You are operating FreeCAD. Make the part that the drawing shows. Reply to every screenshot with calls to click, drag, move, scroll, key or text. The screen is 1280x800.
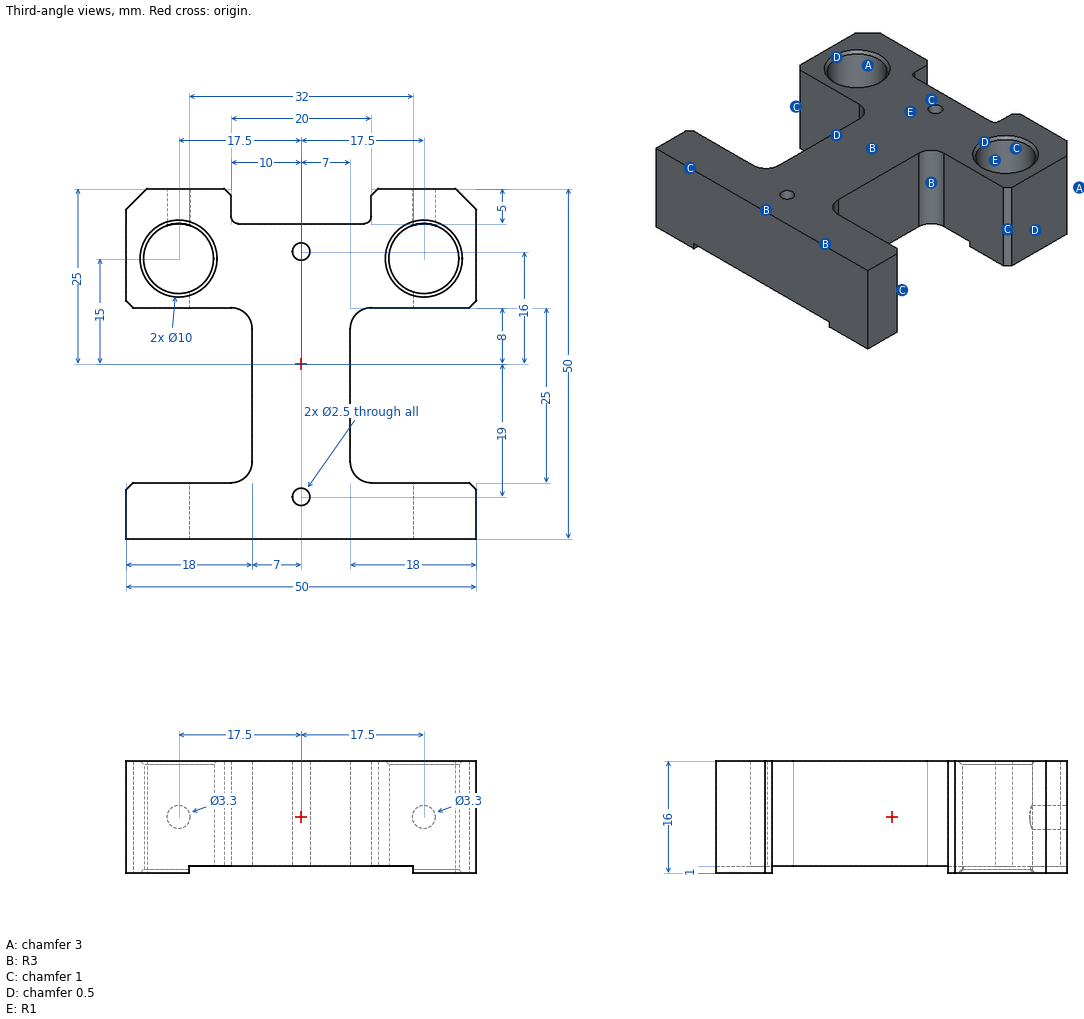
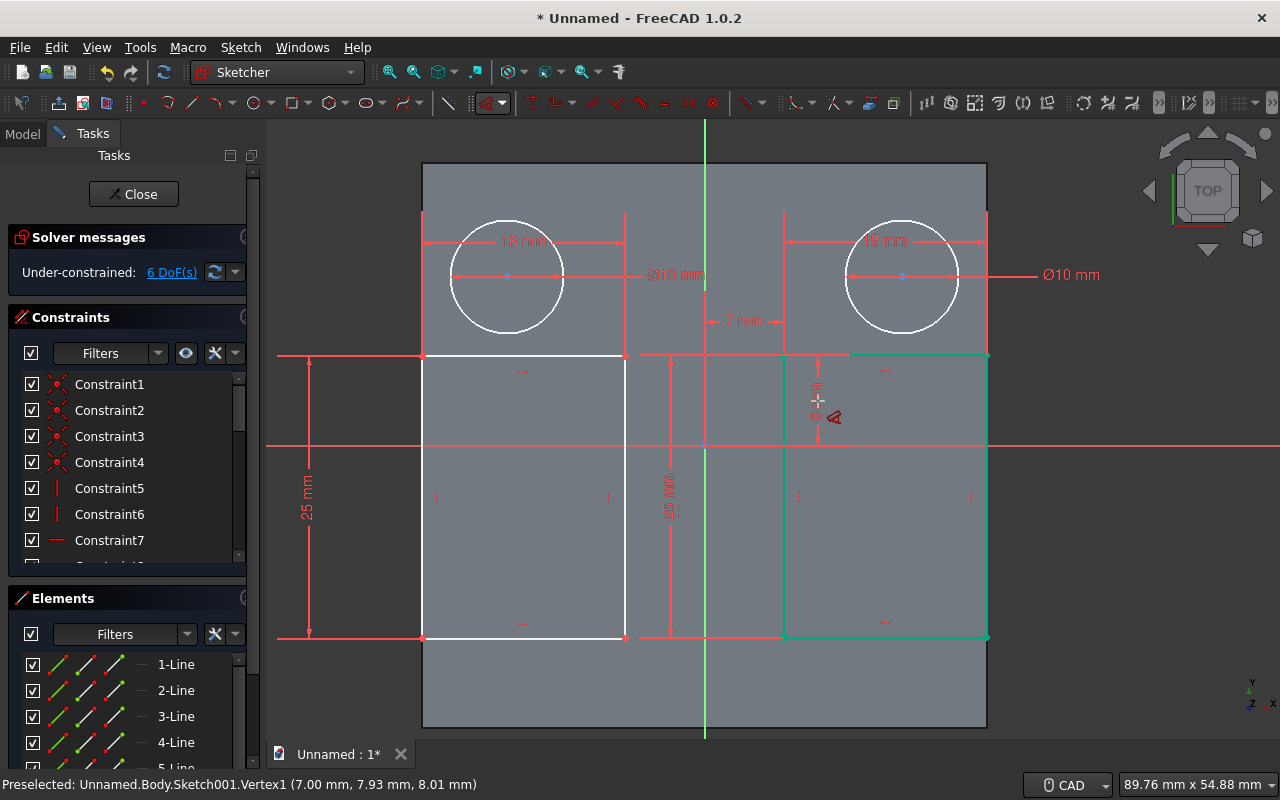
click(422, 356)
click(388, 401)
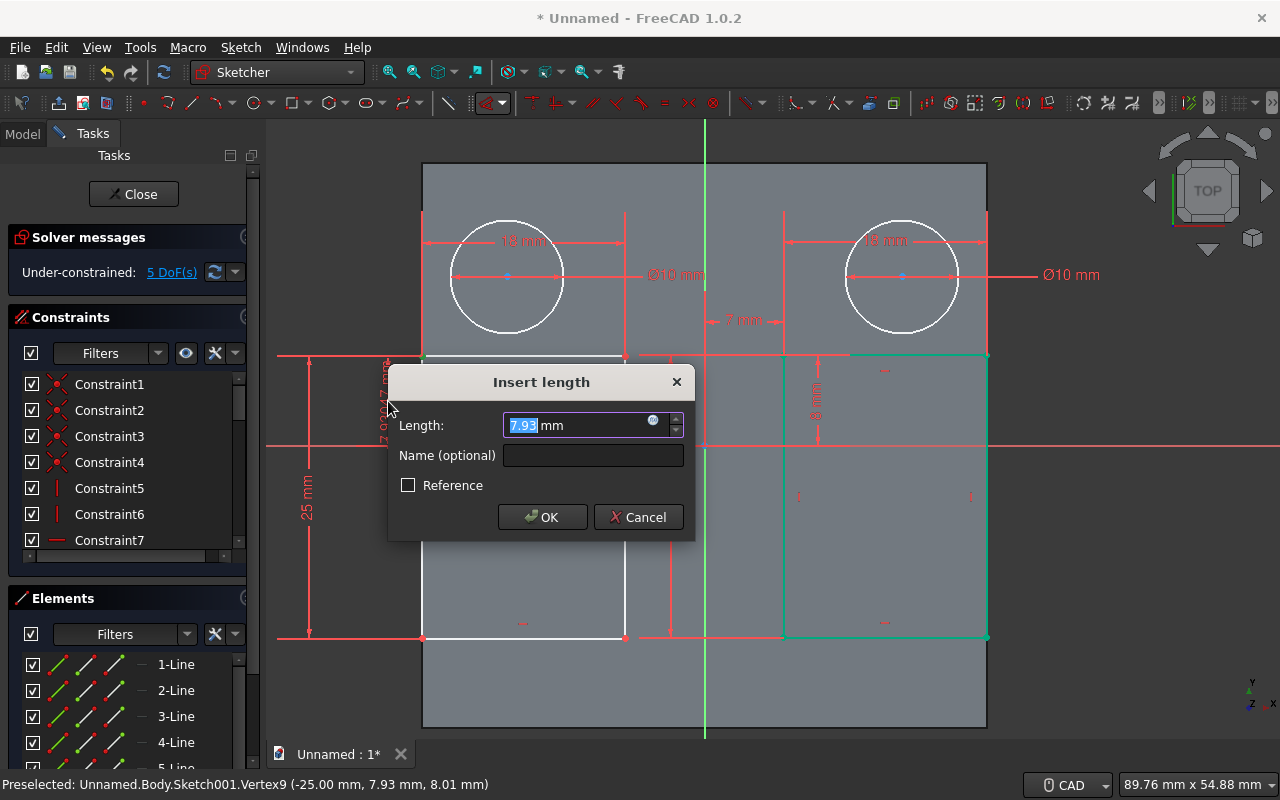
text(8)
key(Return)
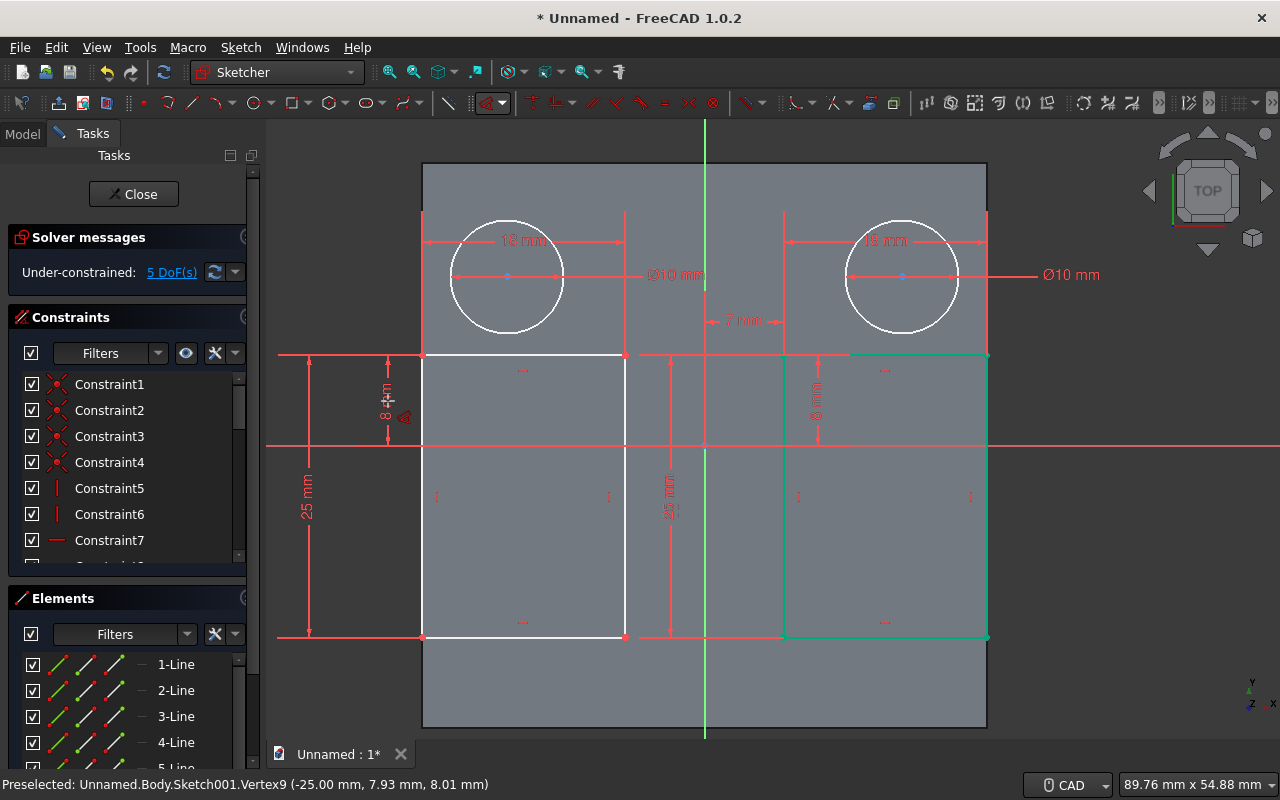
click(625, 638)
click(665, 672)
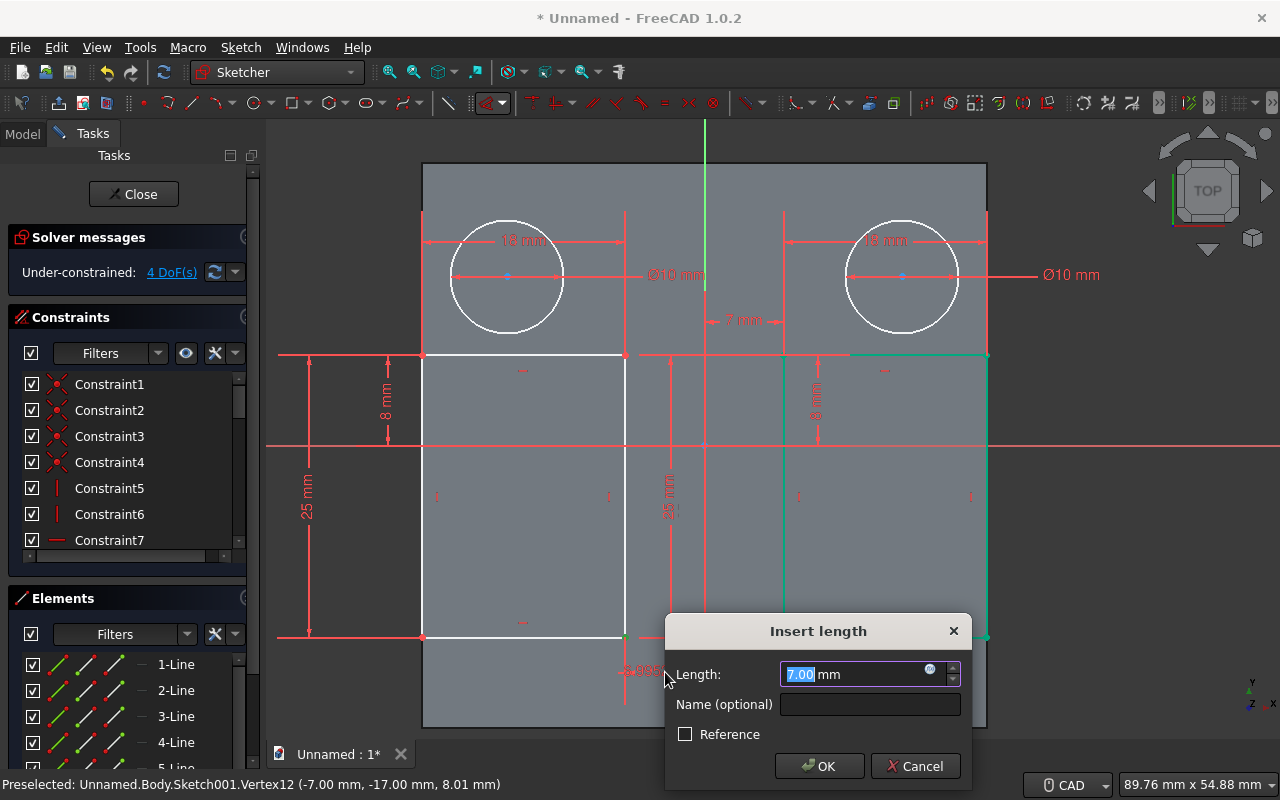
text(7)
key(Return)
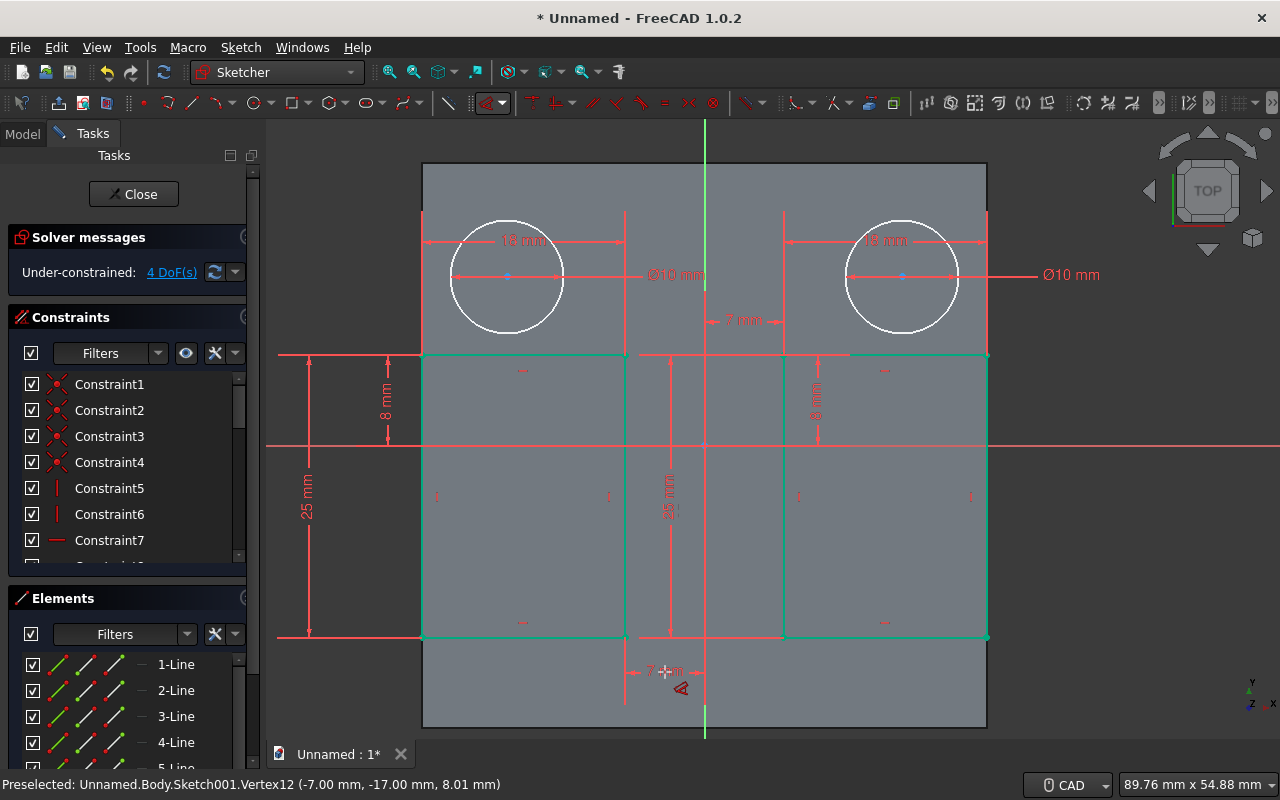
click(507, 277)
click(473, 400)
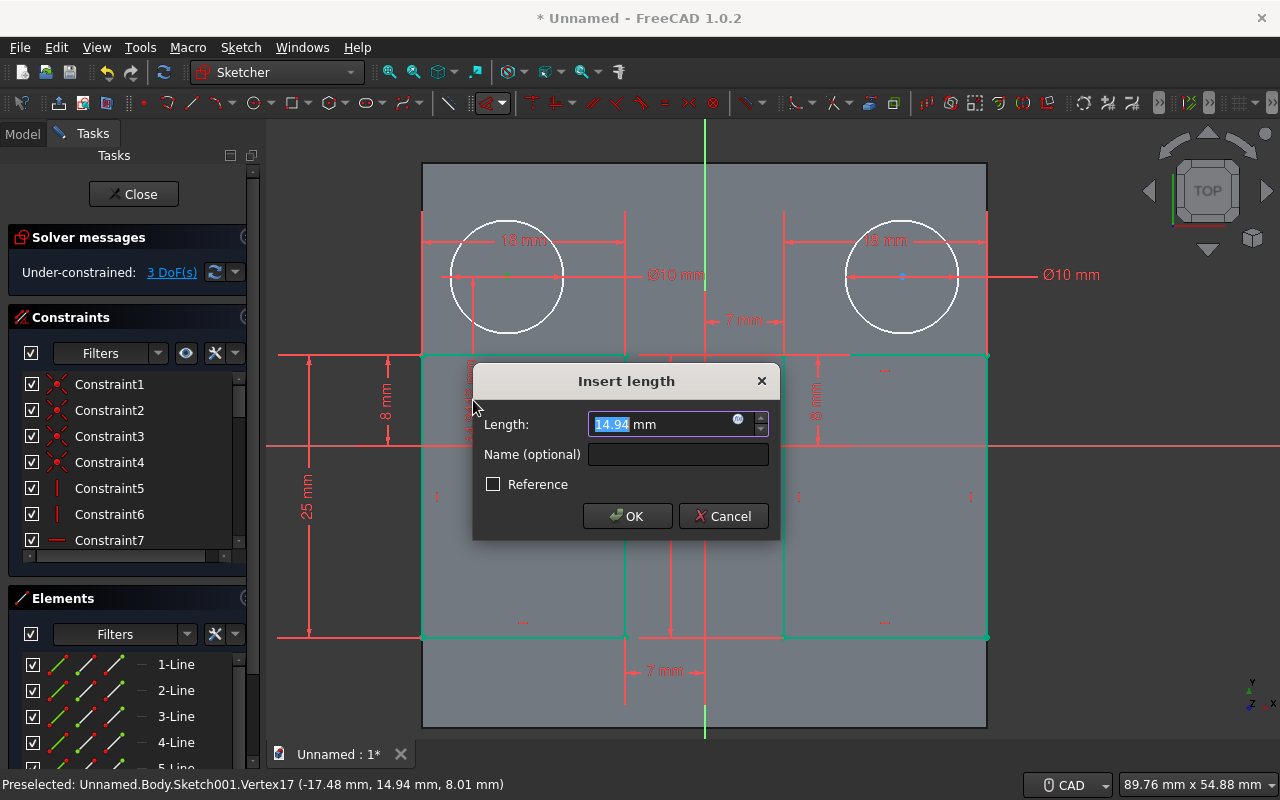
text(15)
key(Return)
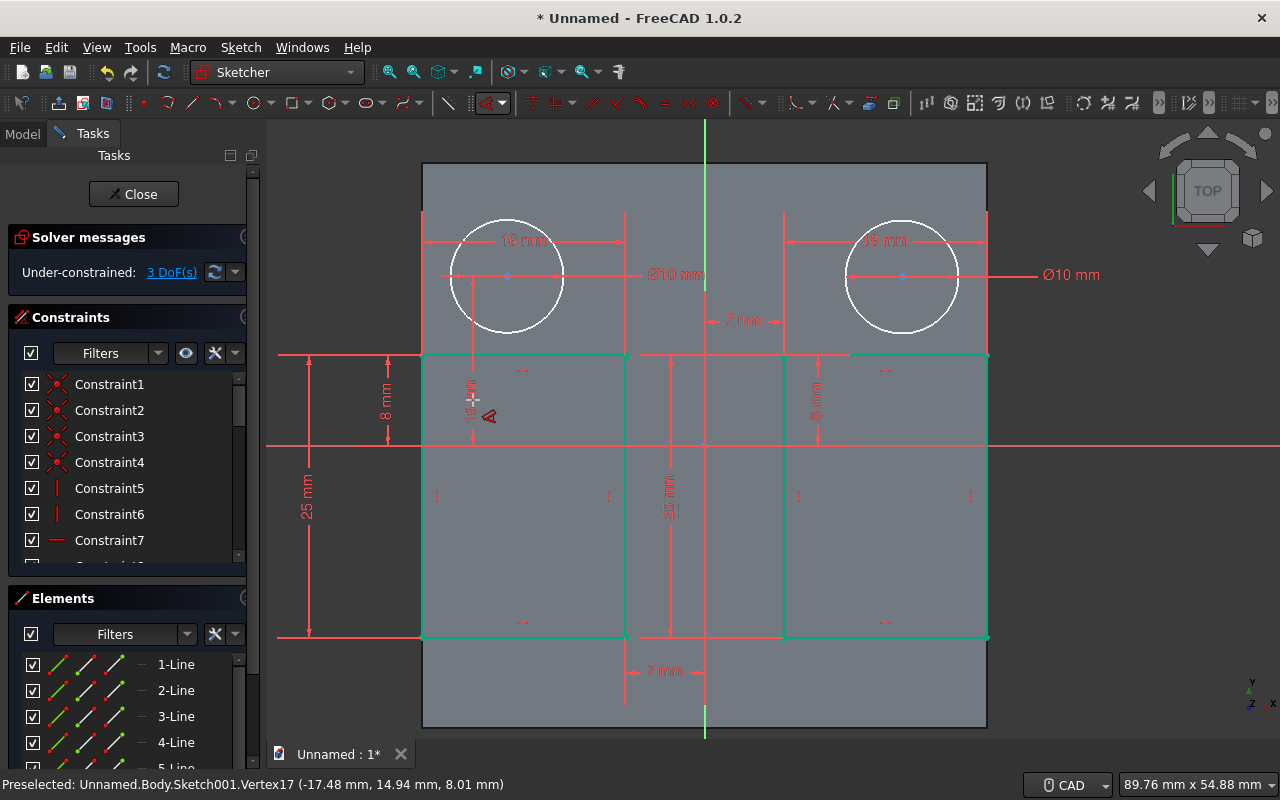
click(902, 277)
click(936, 400)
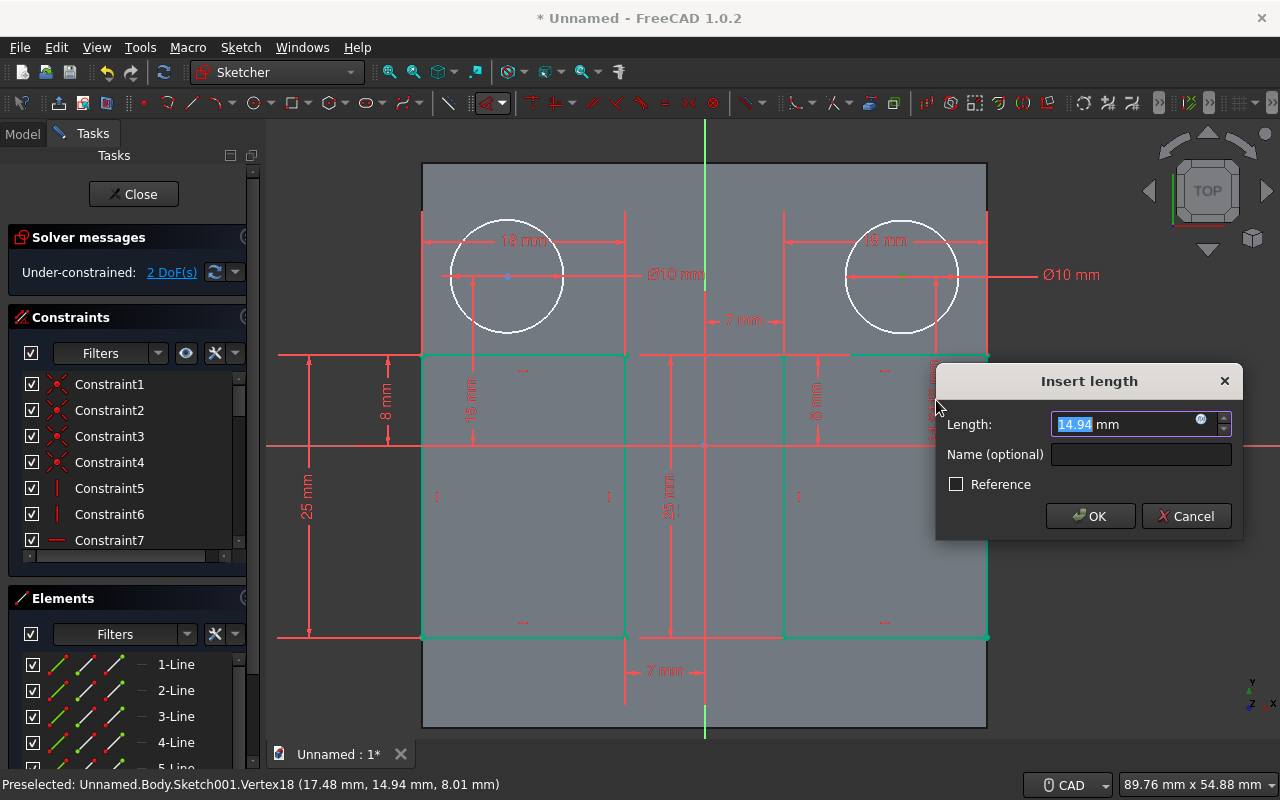
text(15)
key(Return)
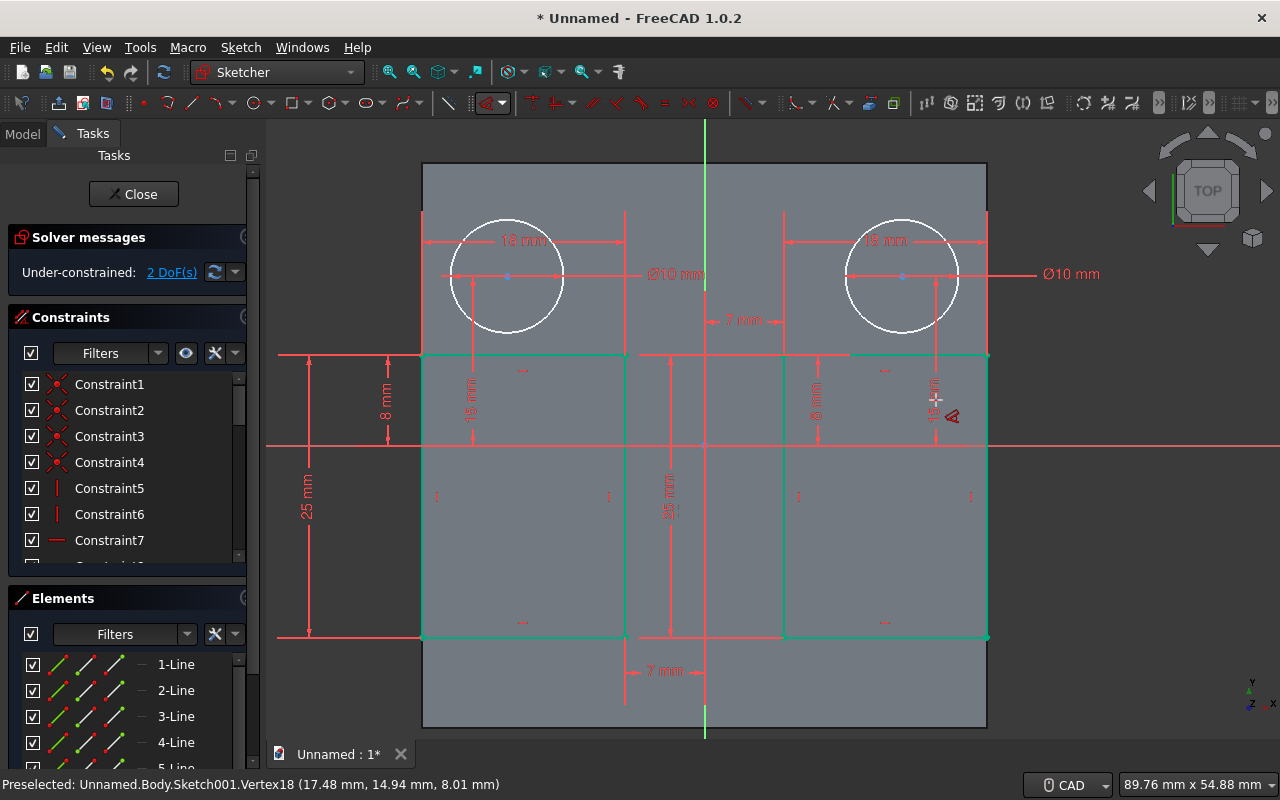
click(507, 276)
click(606, 242)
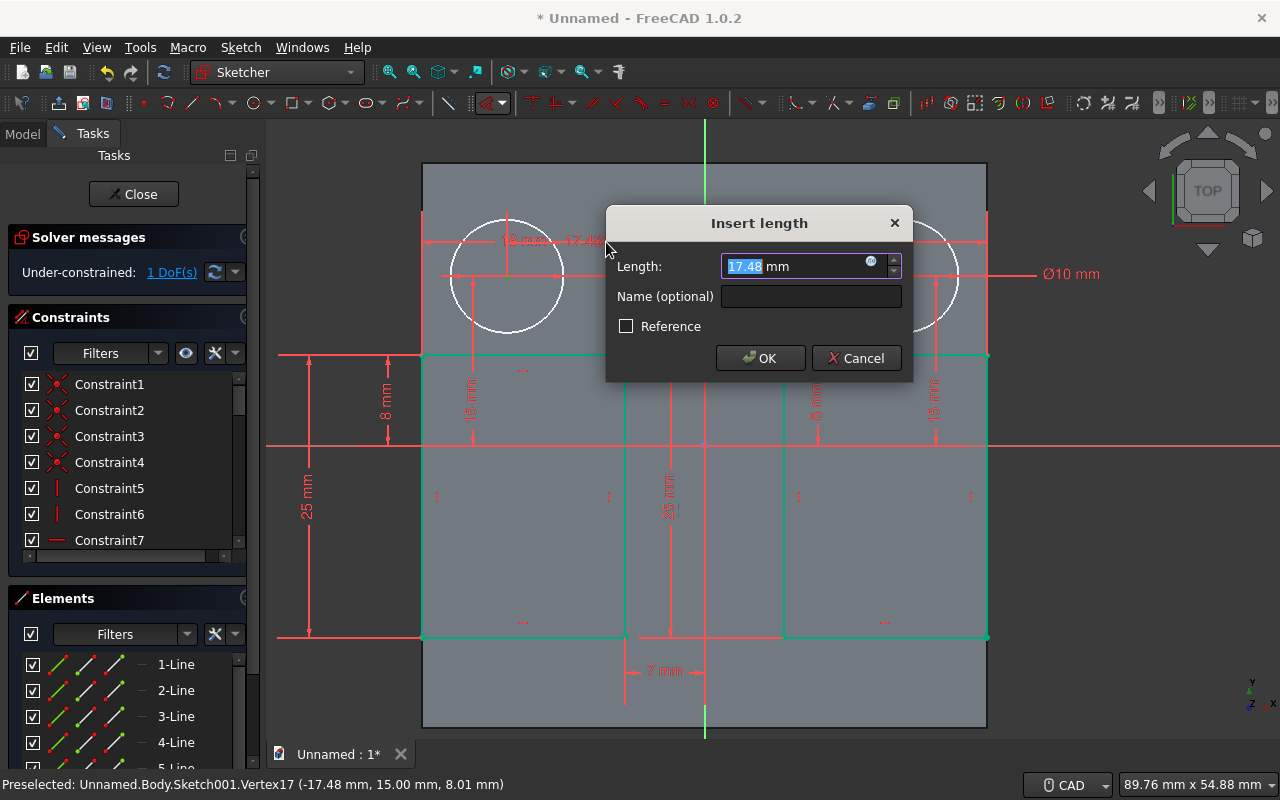
text(17.5)
key(Return)